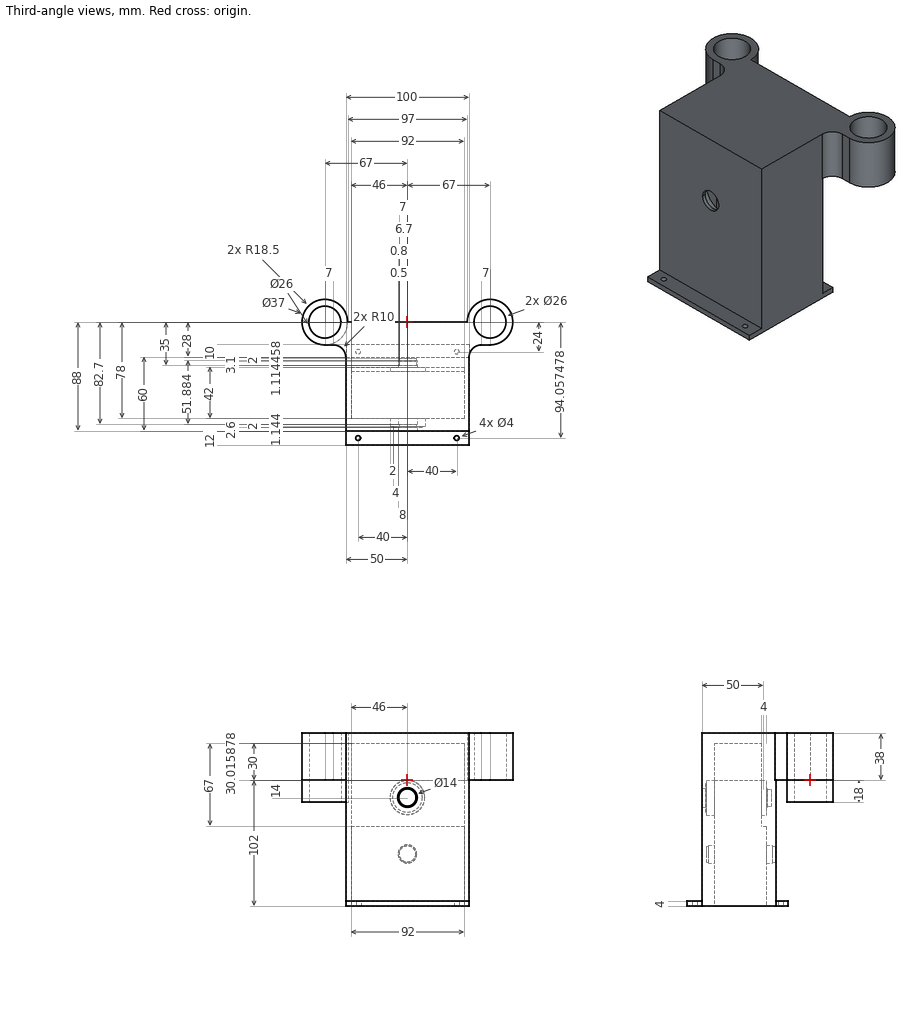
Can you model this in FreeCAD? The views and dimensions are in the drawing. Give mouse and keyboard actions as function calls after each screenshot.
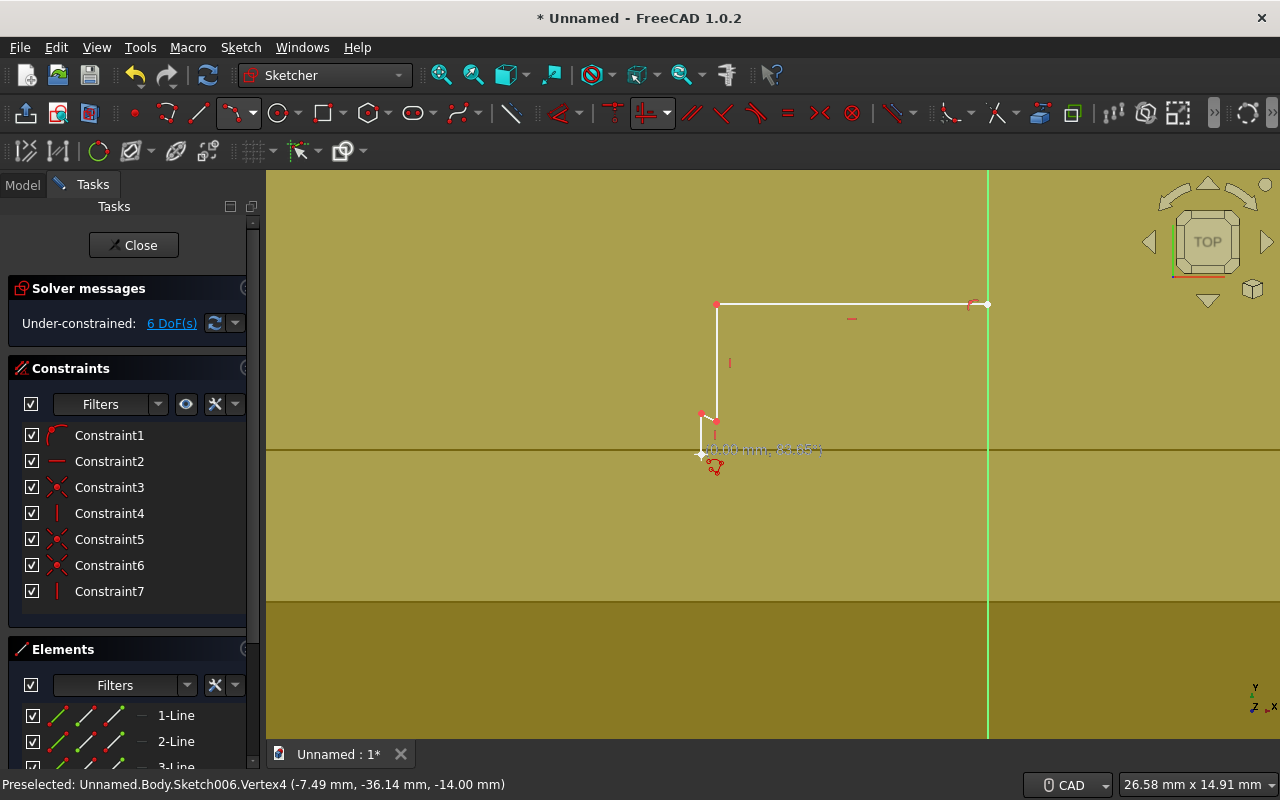
scroll(702, 417, down, 11)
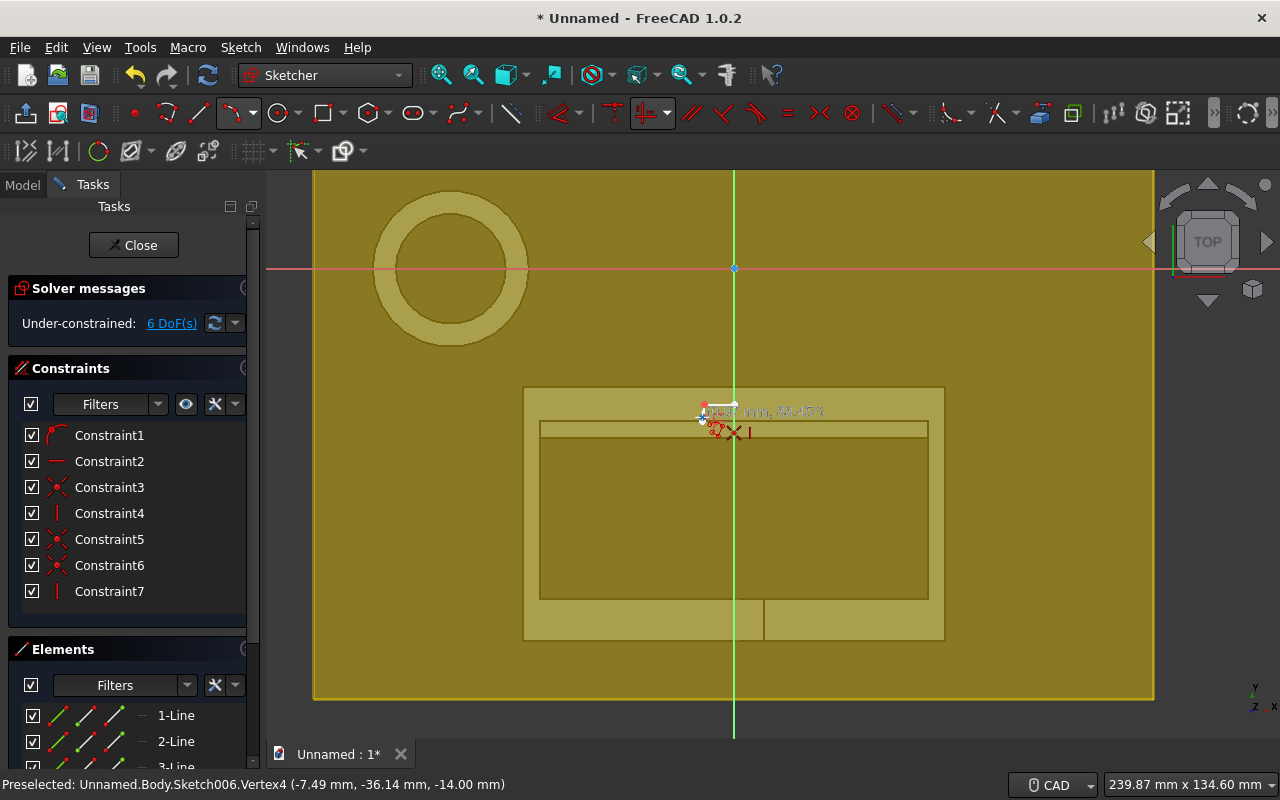
click(675, 421)
click(675, 625)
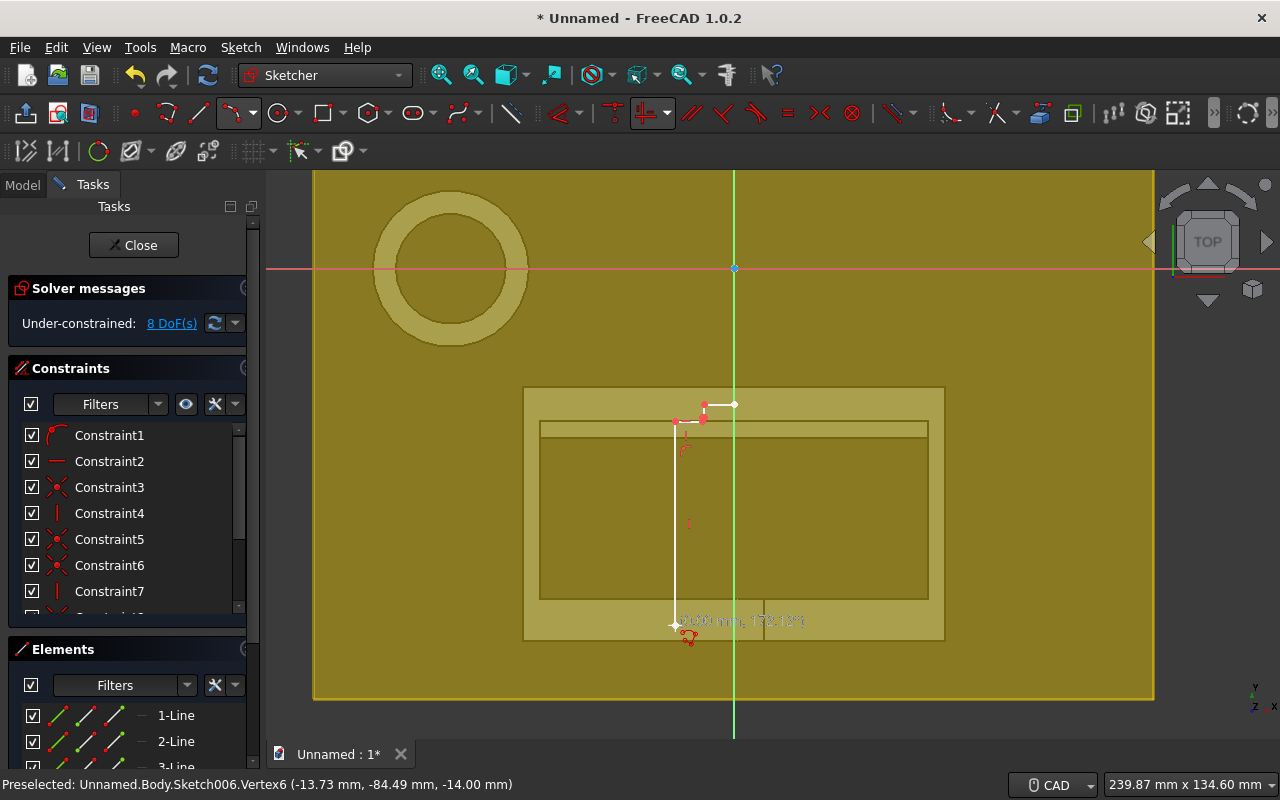
scroll(683, 625, up, 4)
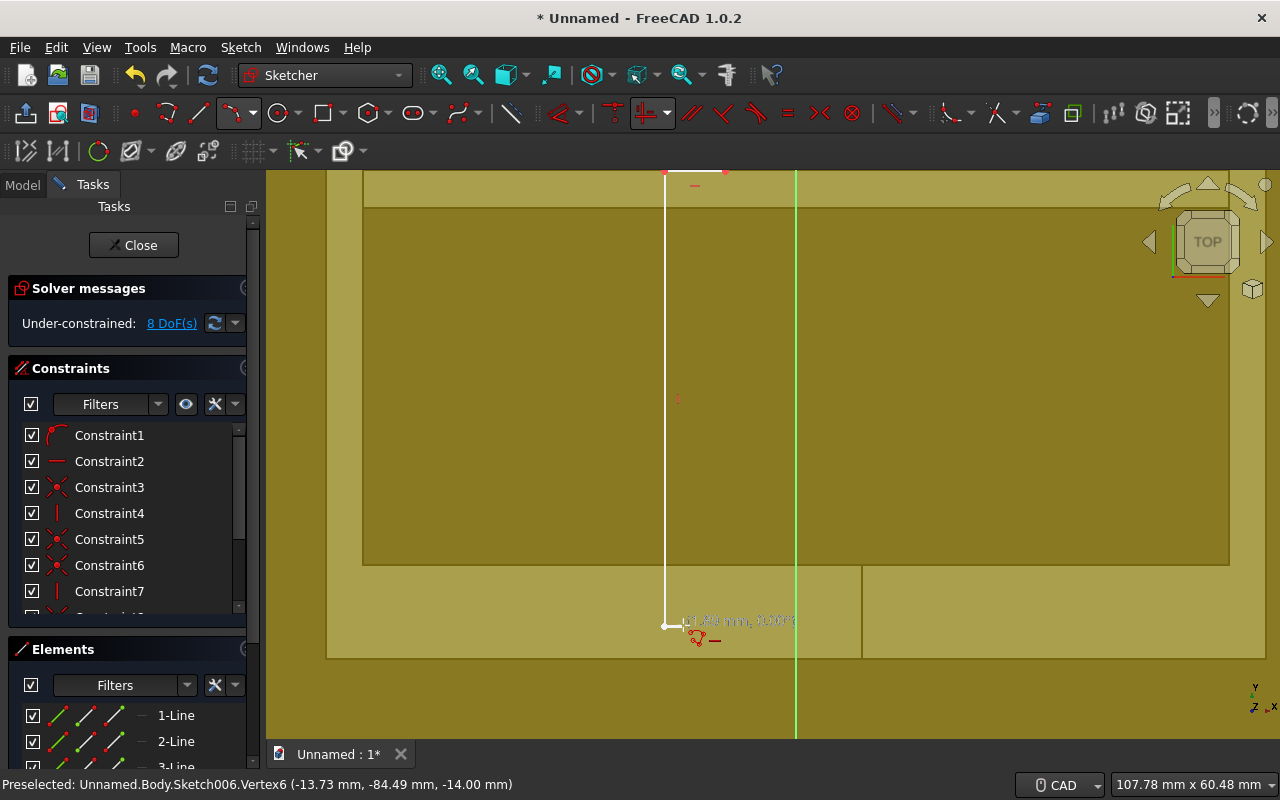
click(683, 624)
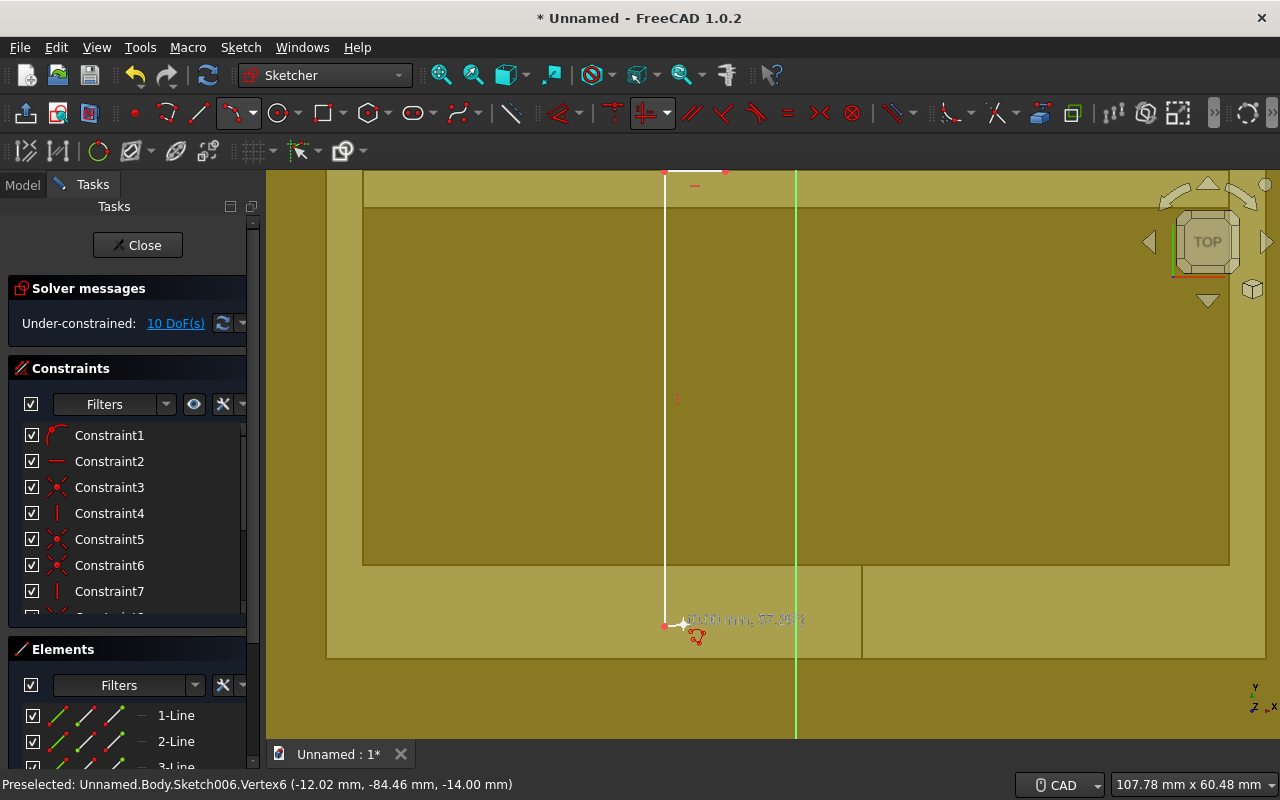
scroll(683, 635, up, 2)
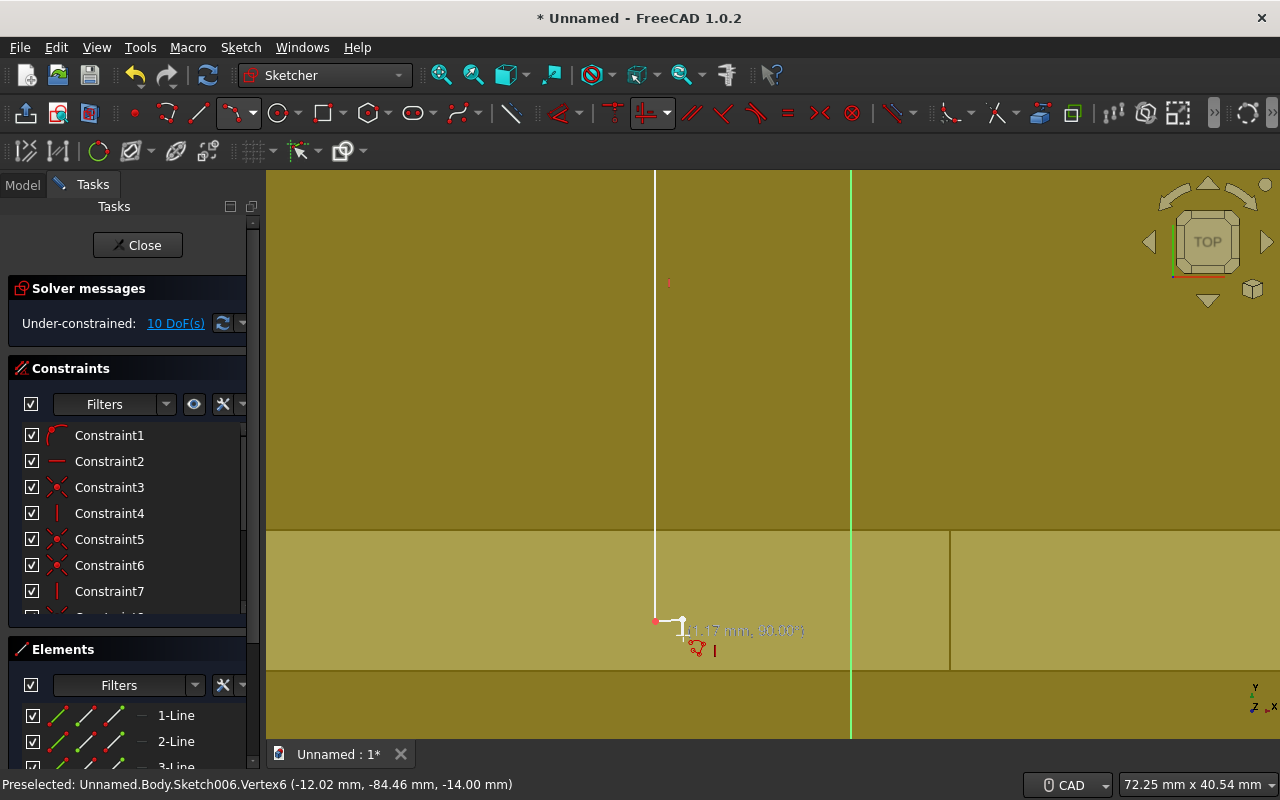
click(683, 634)
click(739, 634)
click(739, 671)
click(842, 671)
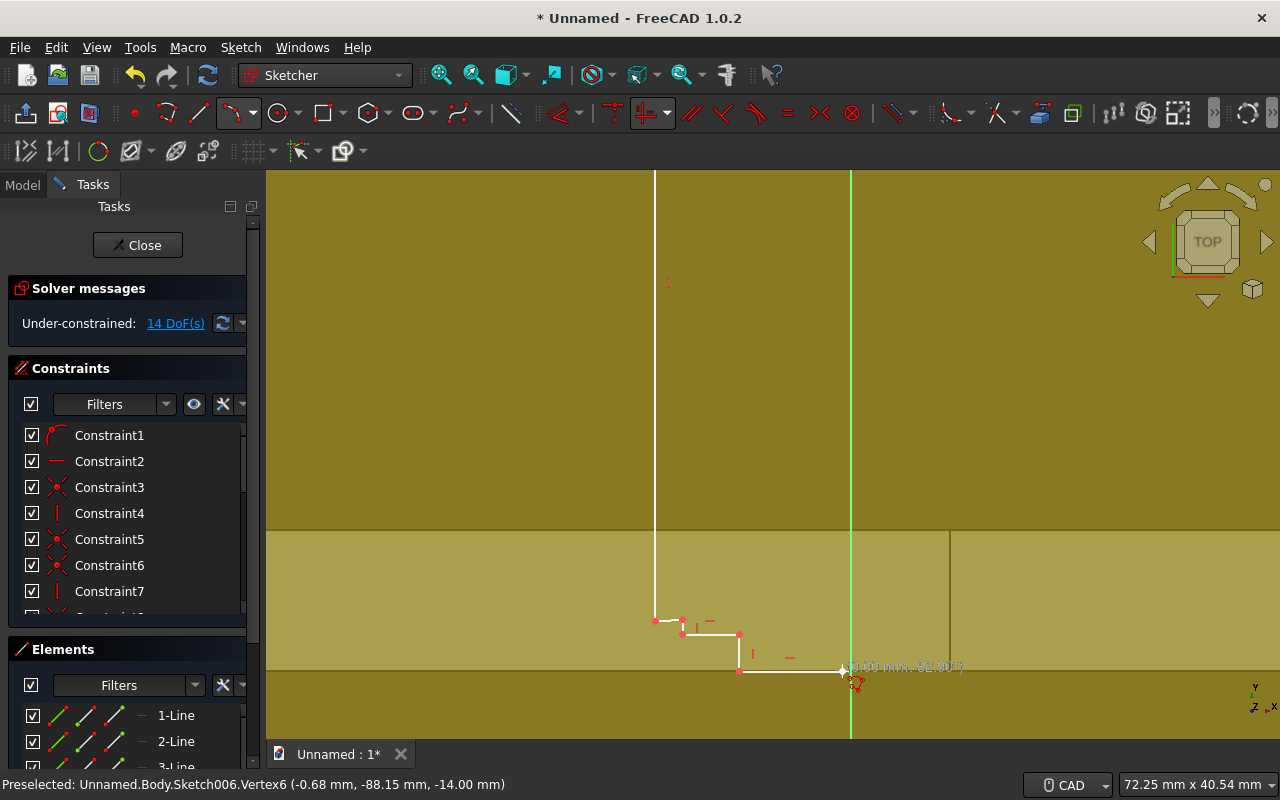
scroll(683, 627, down, 6)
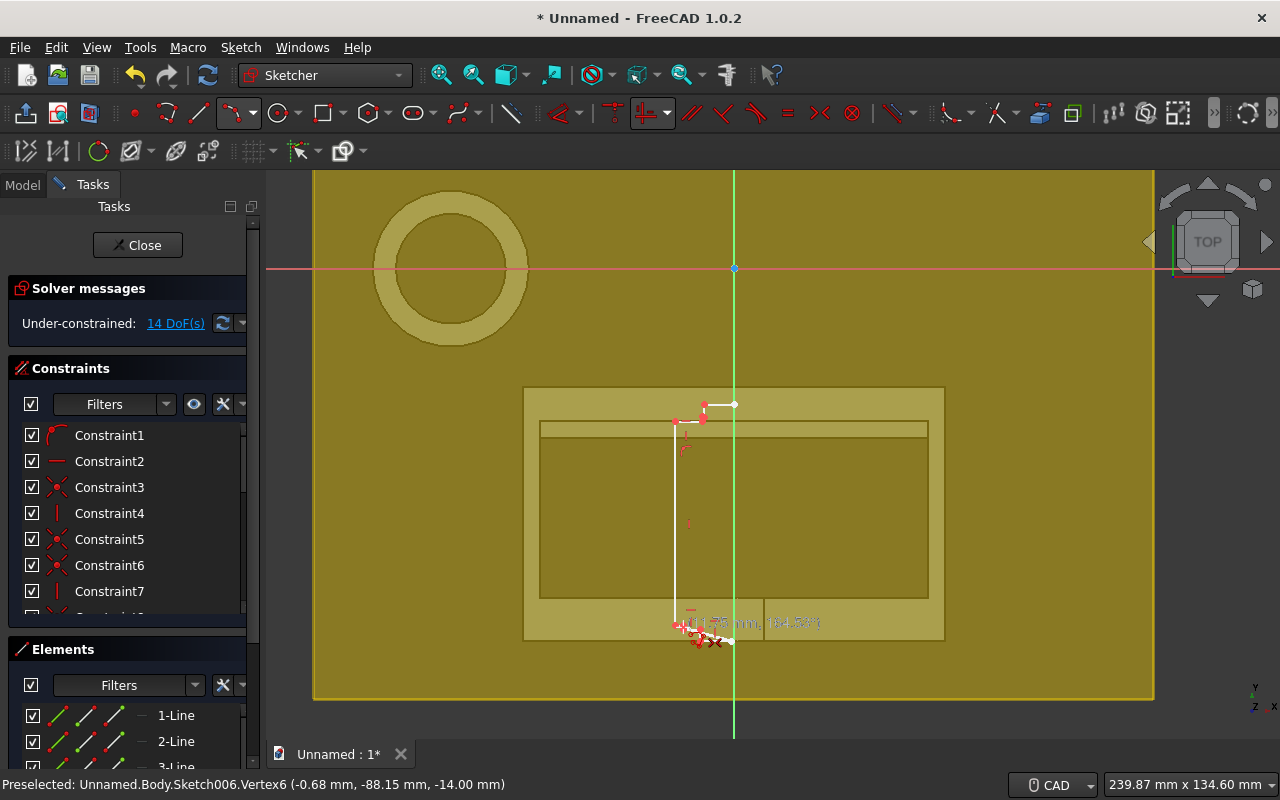
click(734, 405)
key(Escape)
key(Escape)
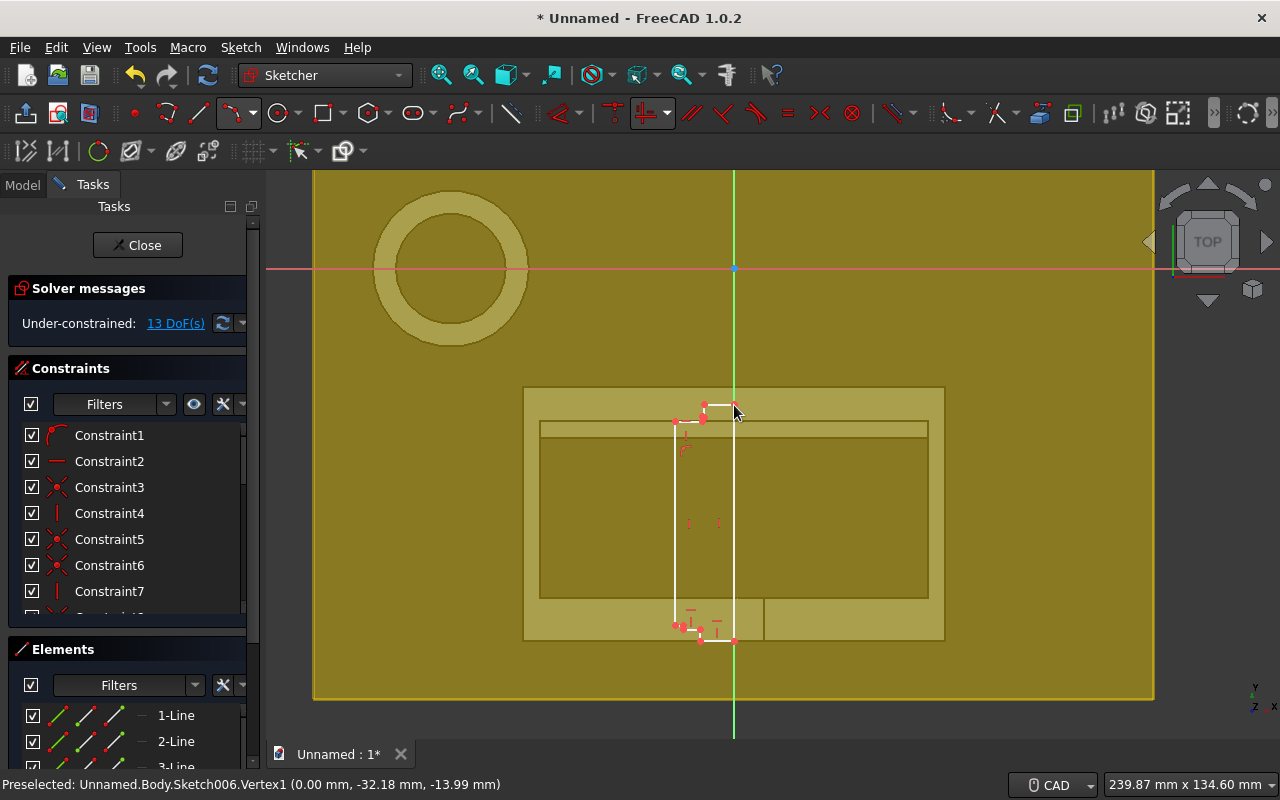
scroll(703, 417, up, 14)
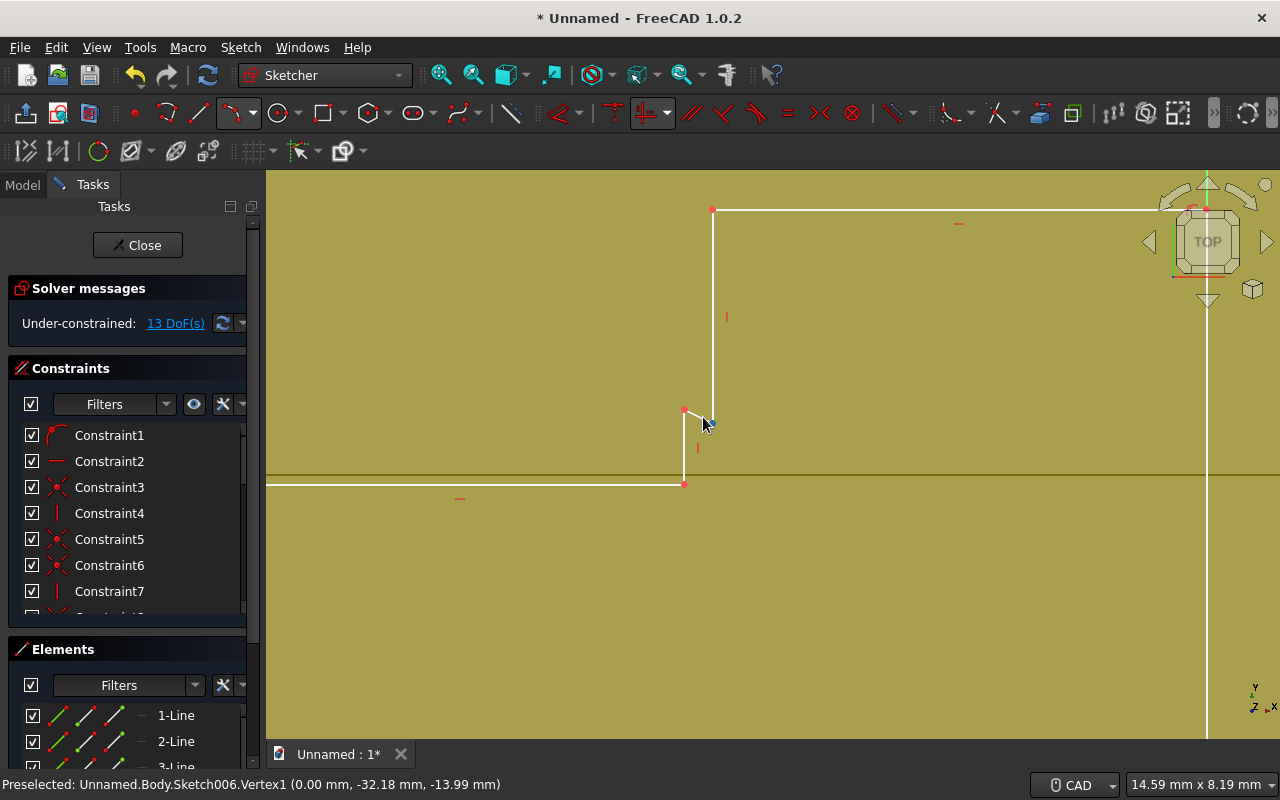
click(699, 417)